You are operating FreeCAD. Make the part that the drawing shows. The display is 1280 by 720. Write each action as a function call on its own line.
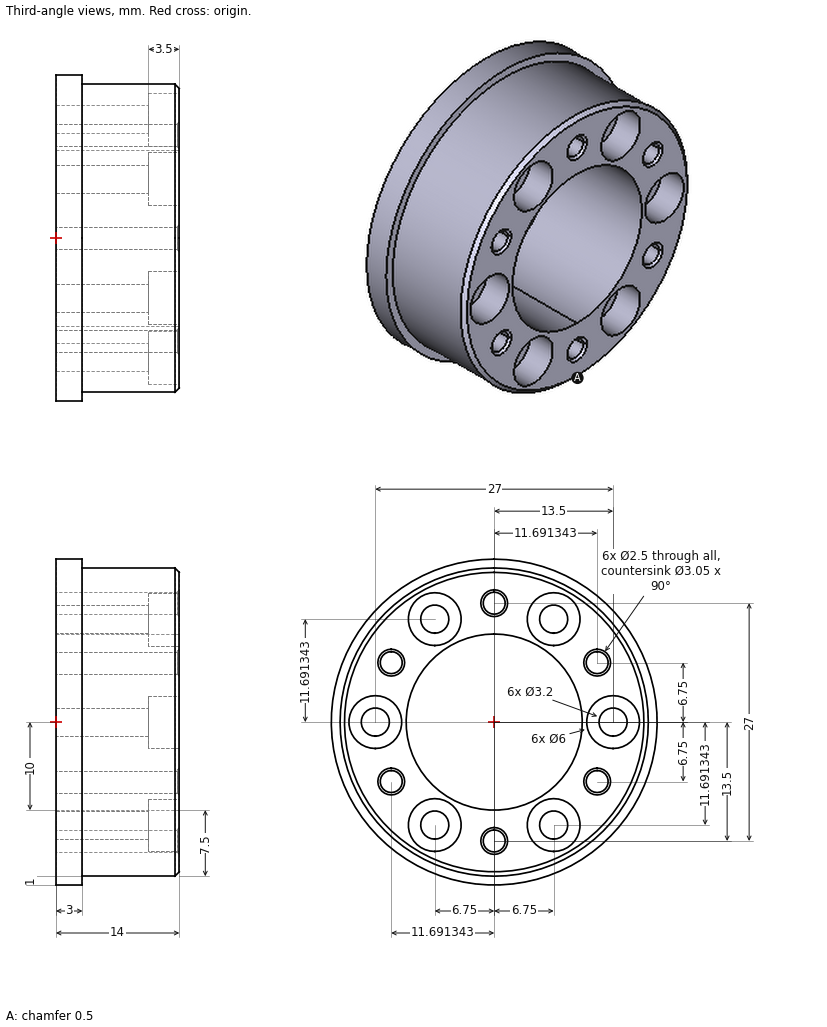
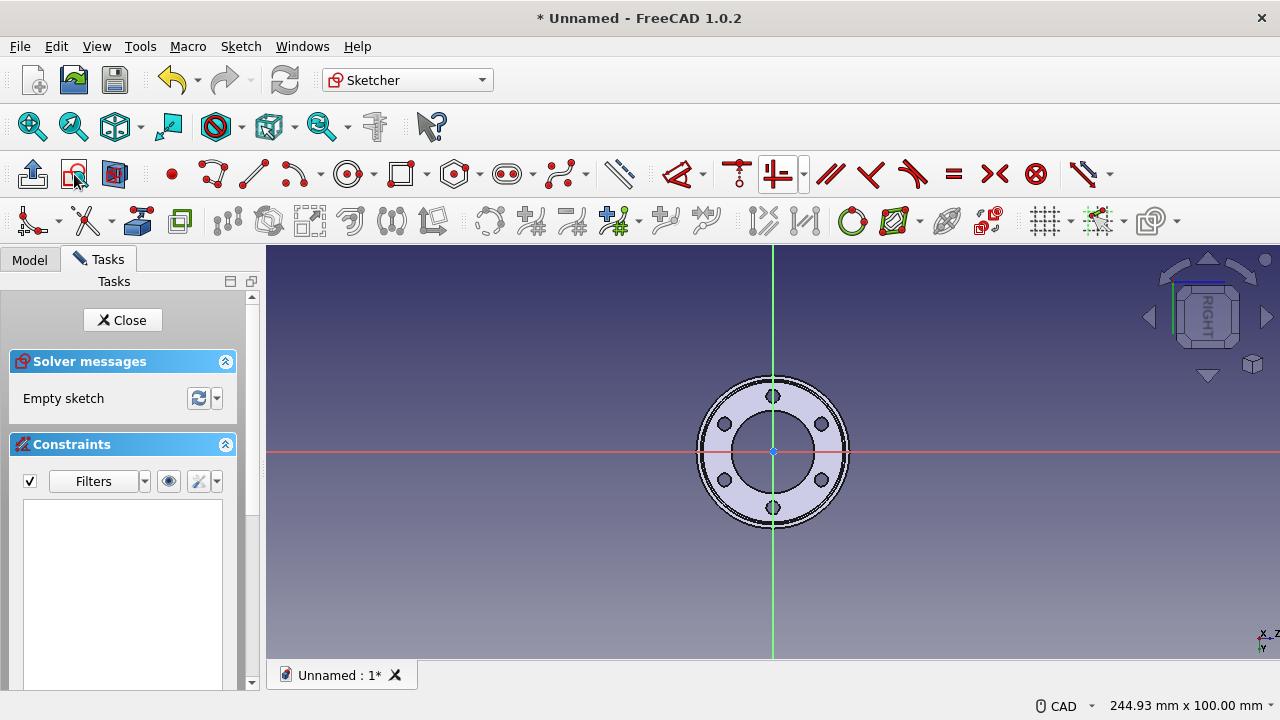
scroll(856, 452, up, 3)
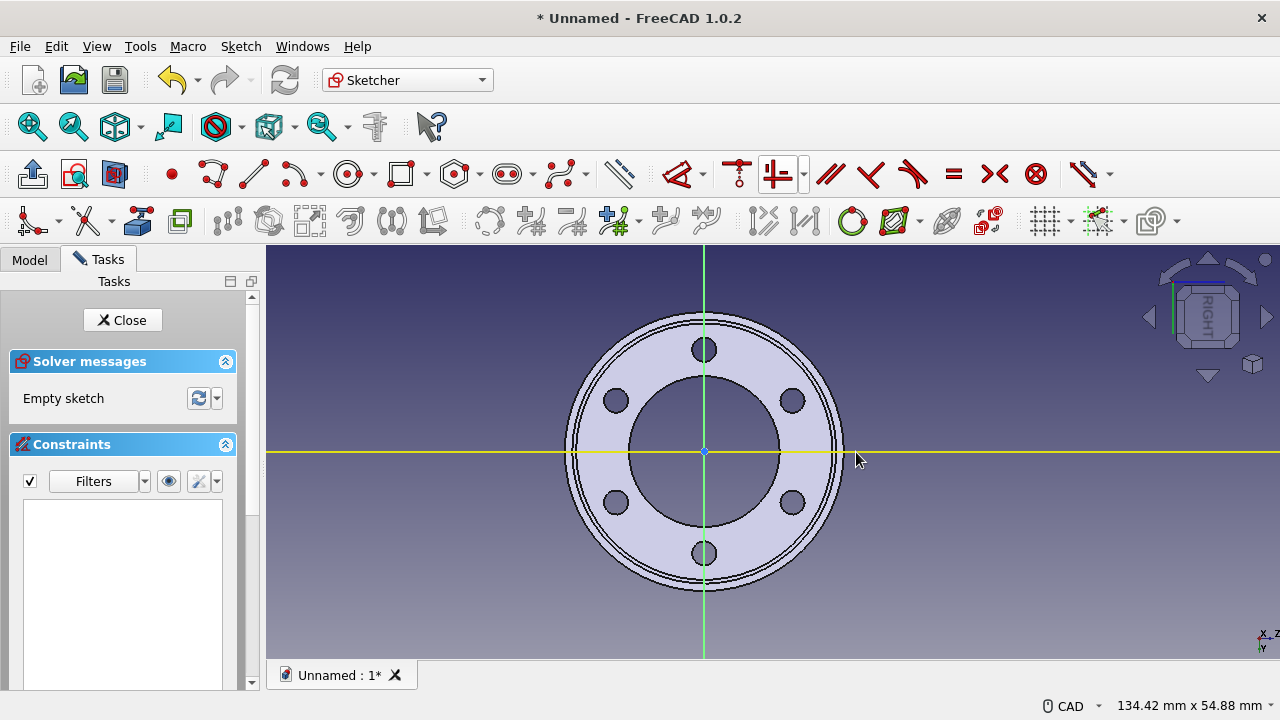
click(348, 174)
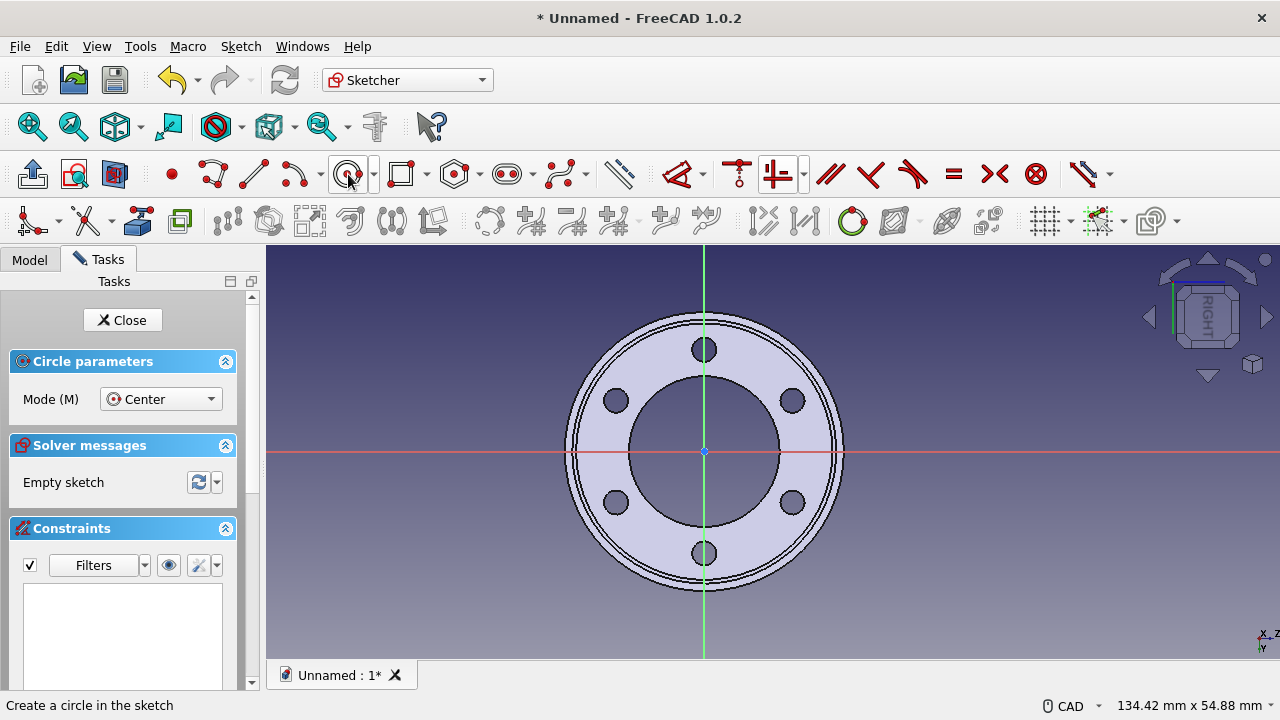
click(704, 553)
click(720, 537)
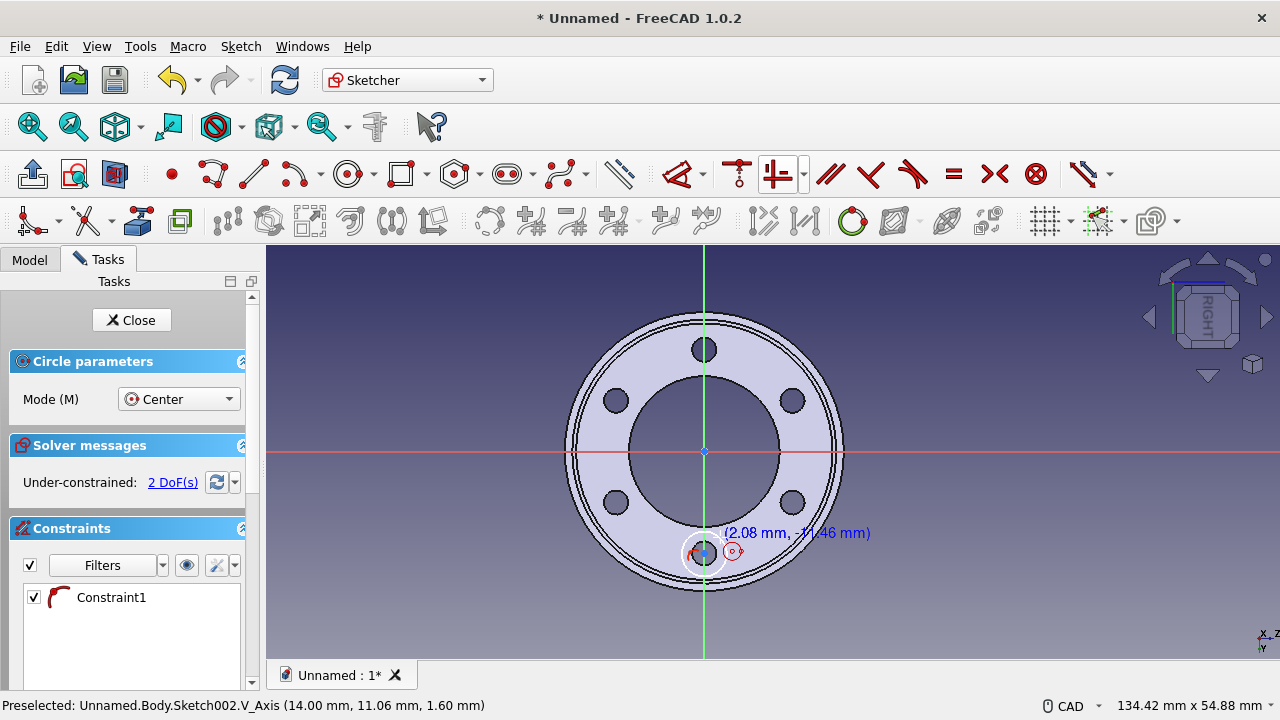
click(616, 503)
click(632, 487)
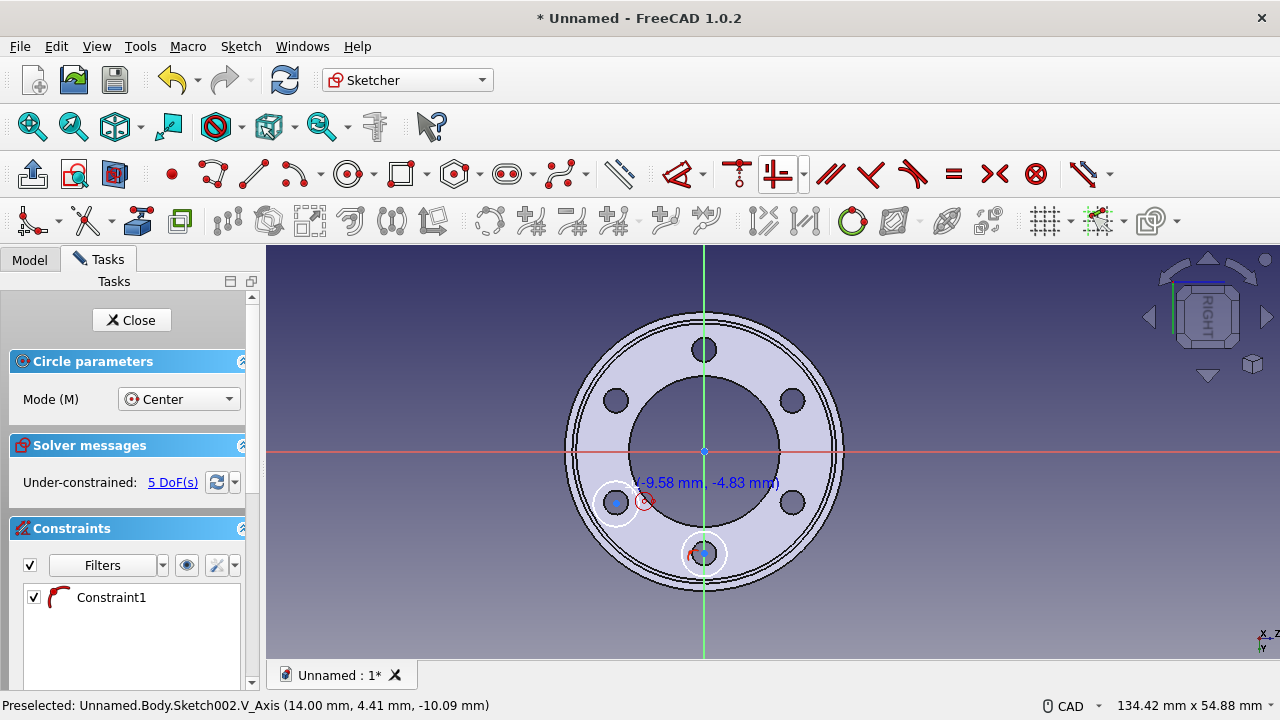
click(616, 401)
click(632, 385)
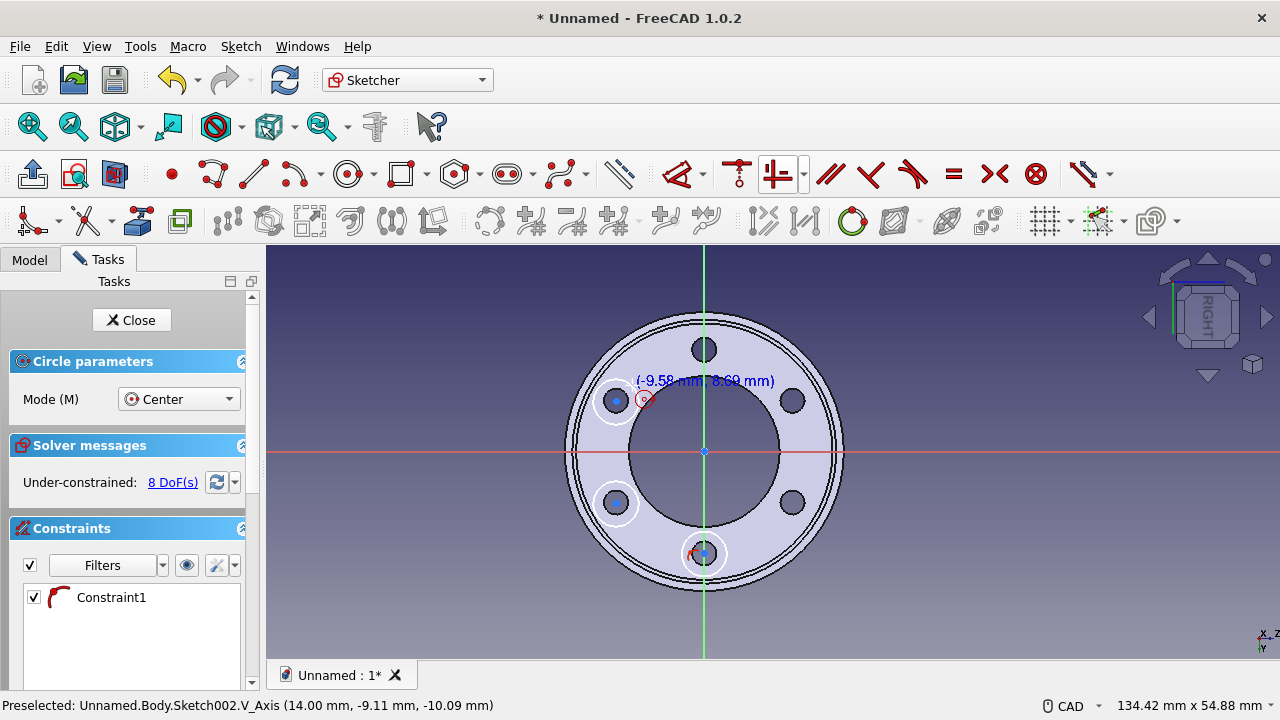
click(704, 350)
click(720, 334)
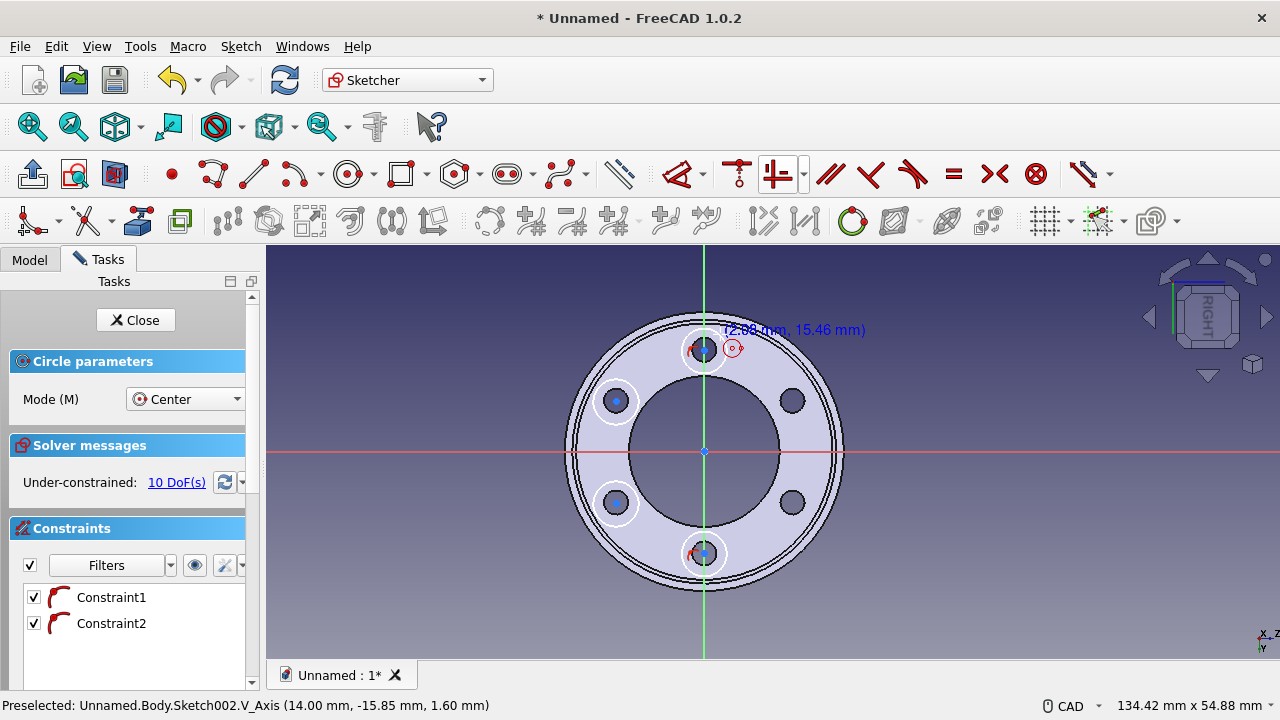
click(792, 401)
click(808, 385)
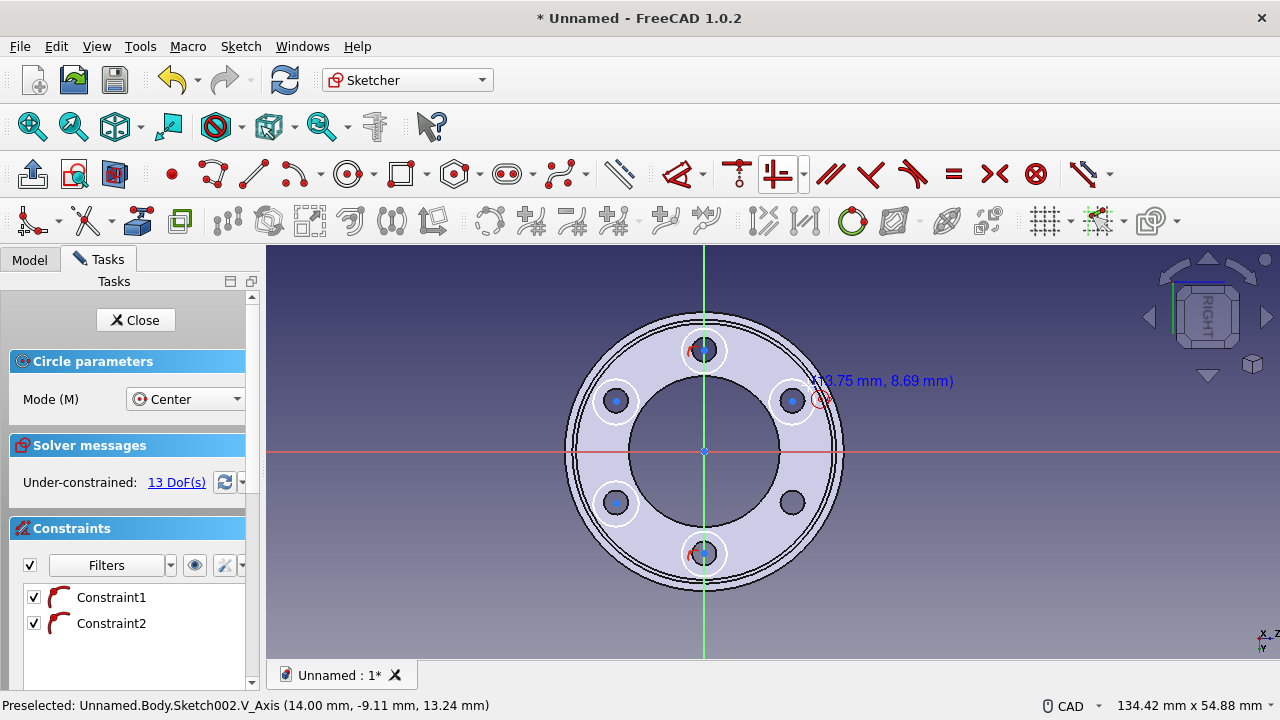
click(792, 503)
click(808, 487)
key(Escape)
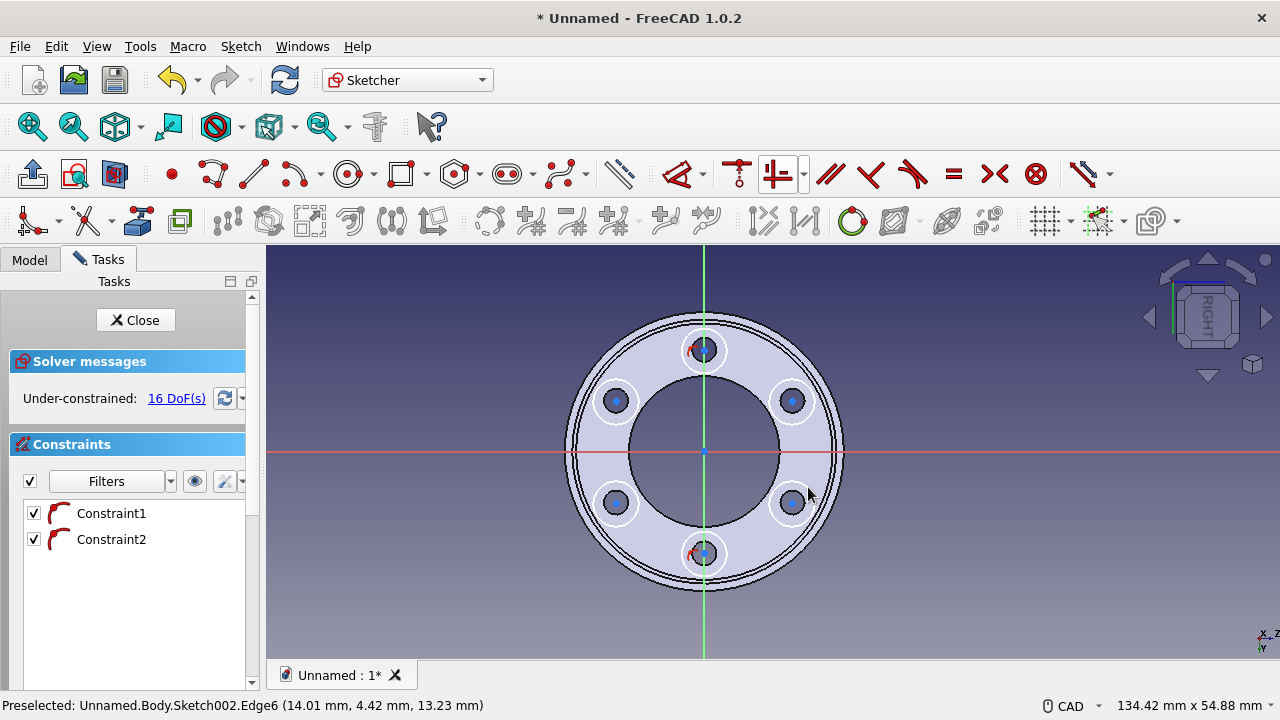
click(720, 538)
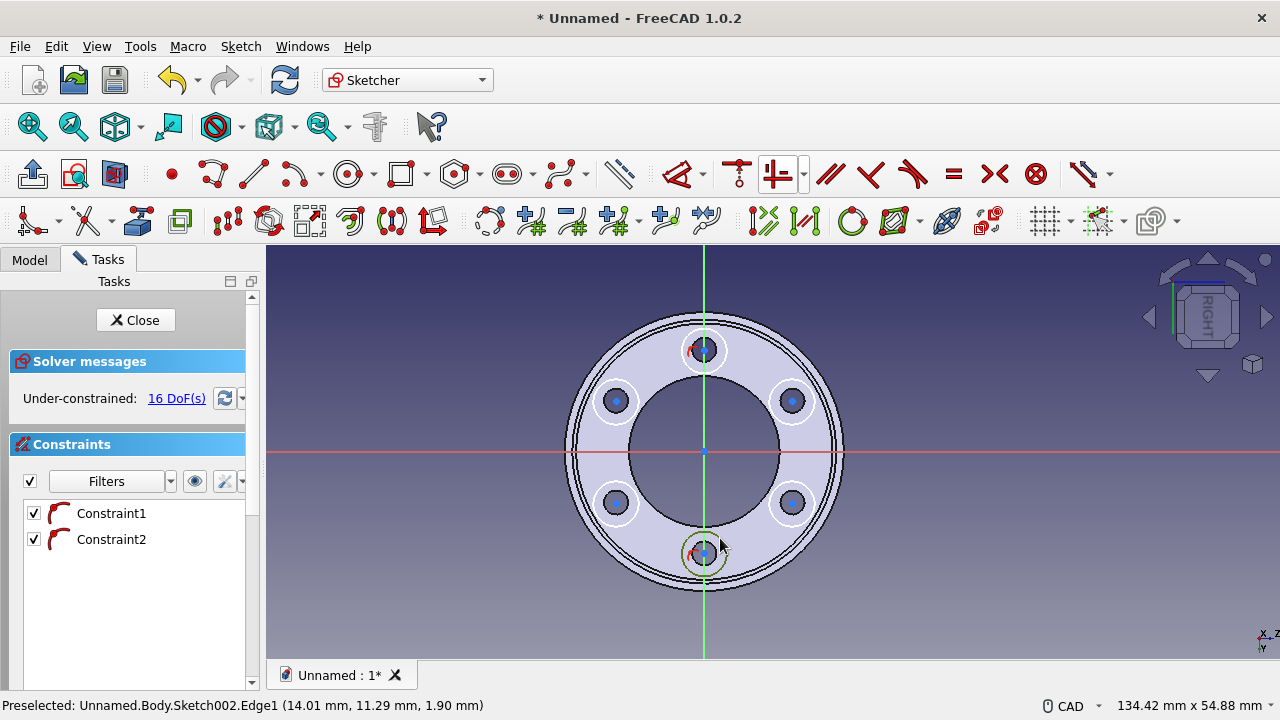
click(632, 488)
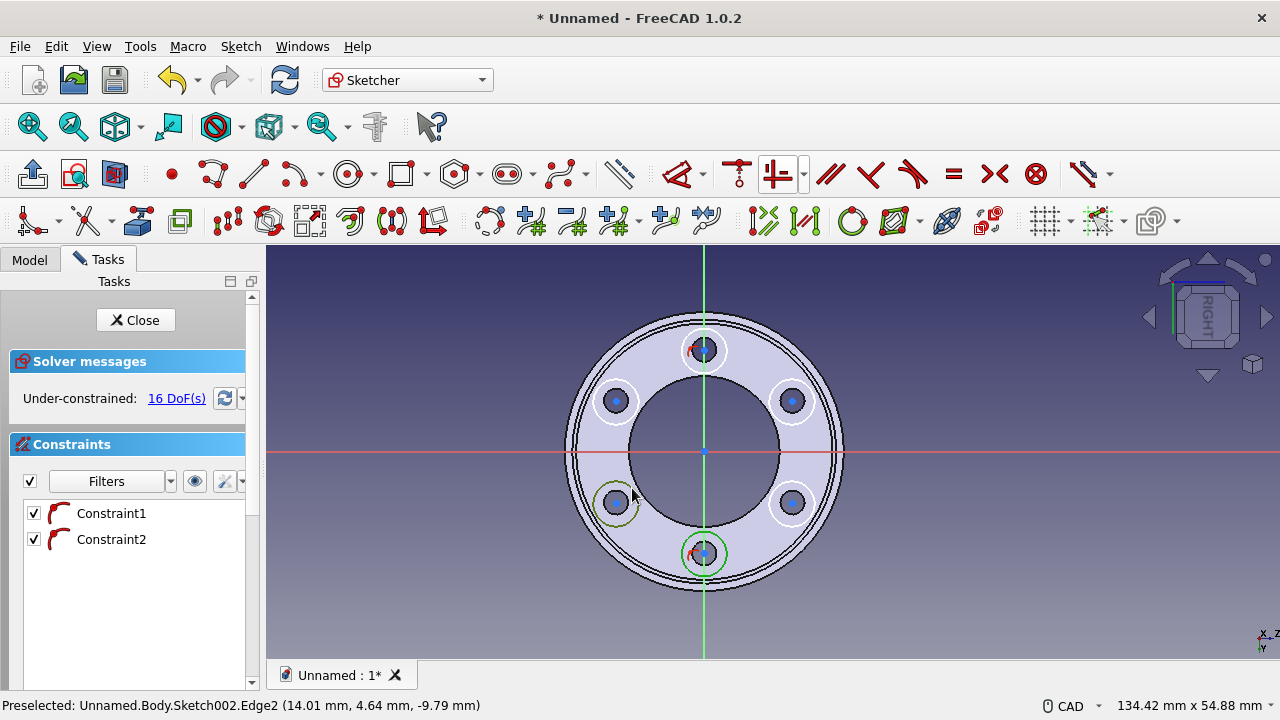
click(632, 386)